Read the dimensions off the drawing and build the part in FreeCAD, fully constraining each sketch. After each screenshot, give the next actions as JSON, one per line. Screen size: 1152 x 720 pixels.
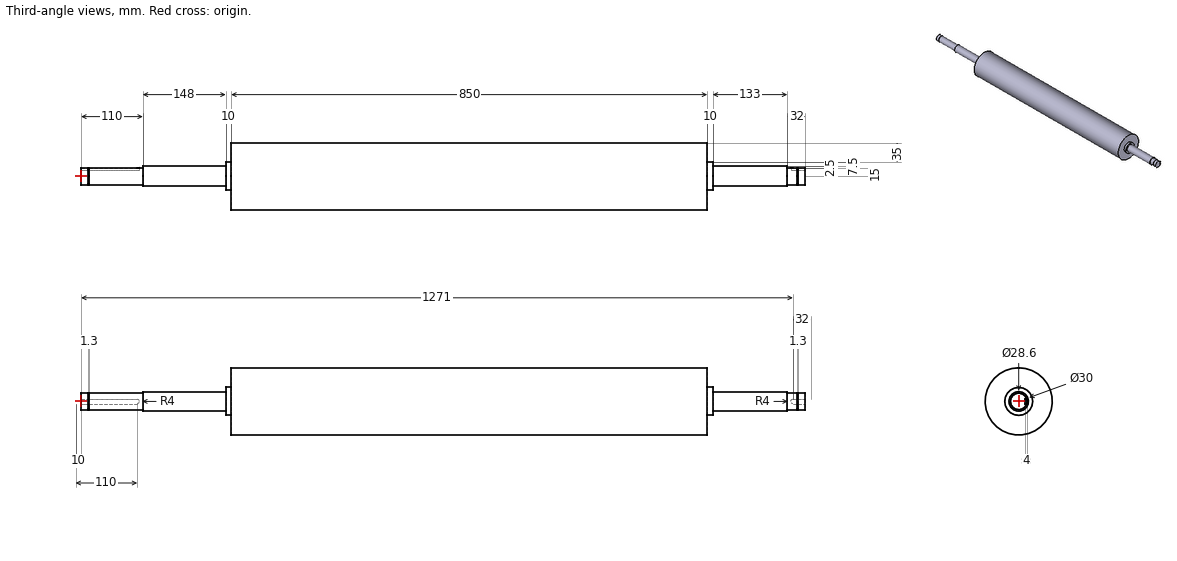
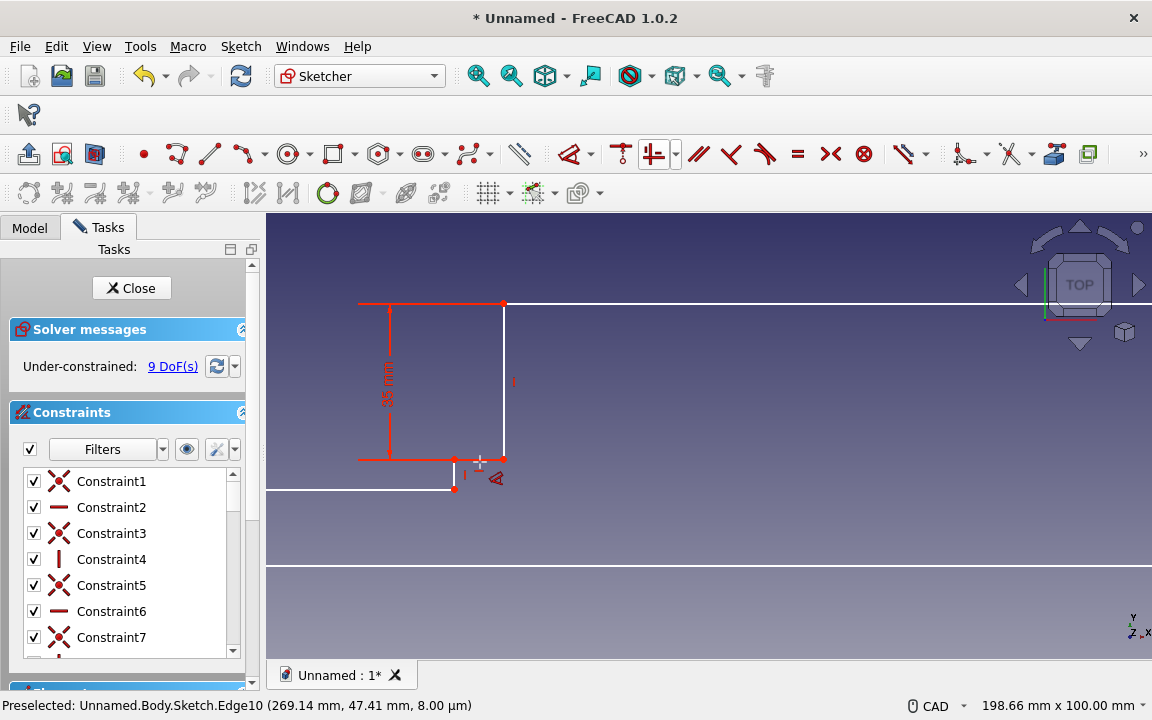
{"action": "left_click", "coordinate": [479, 460]}
{"action": "left_click", "coordinate": [479, 494]}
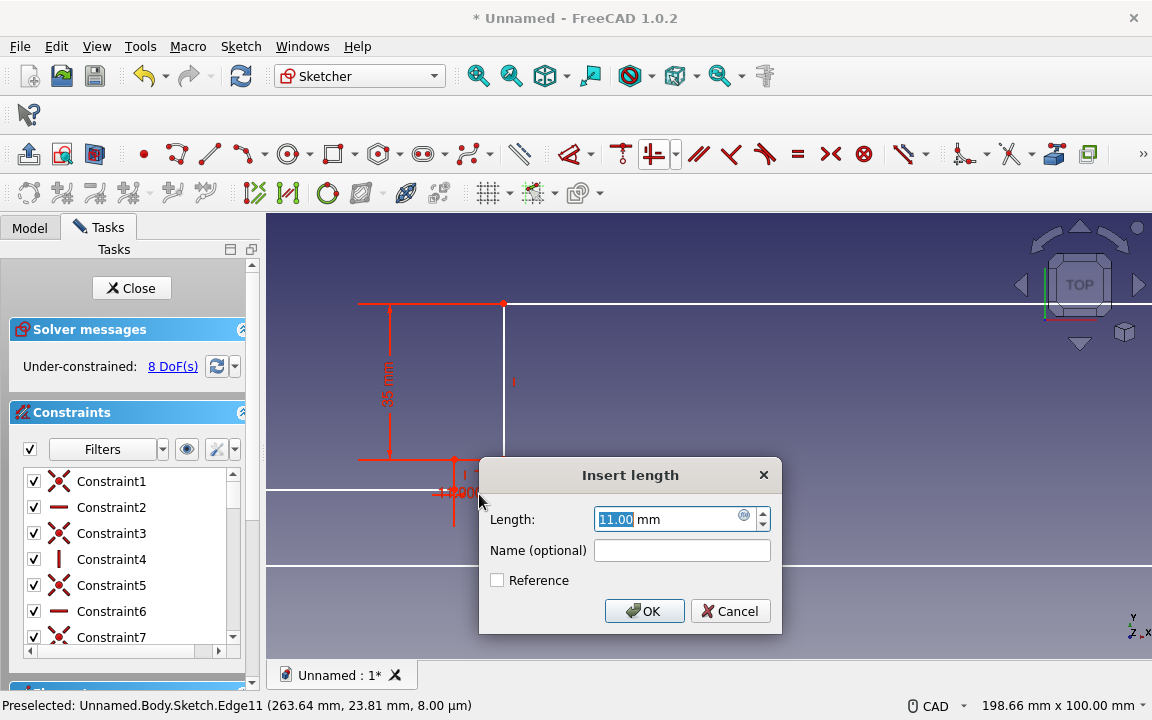
{"action": "type", "text": "10"}
{"action": "key", "text": "Return"}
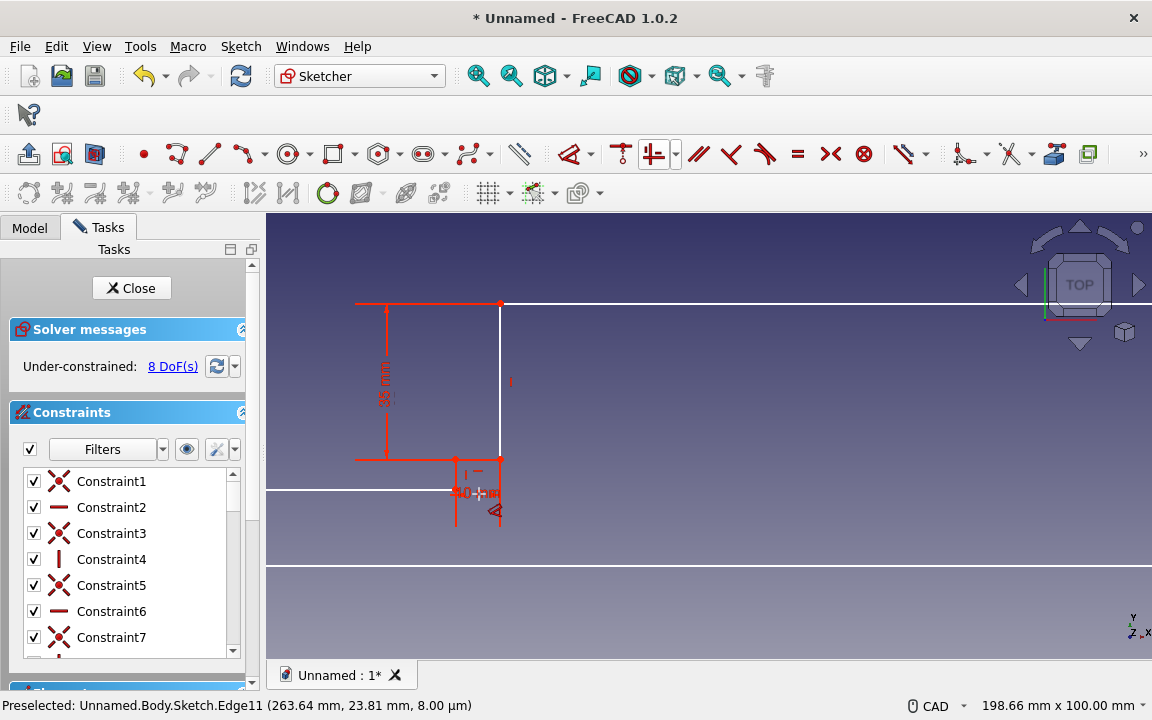
{"action": "scroll", "coordinate": [486, 436], "scroll_direction": "down", "scroll_amount": 12}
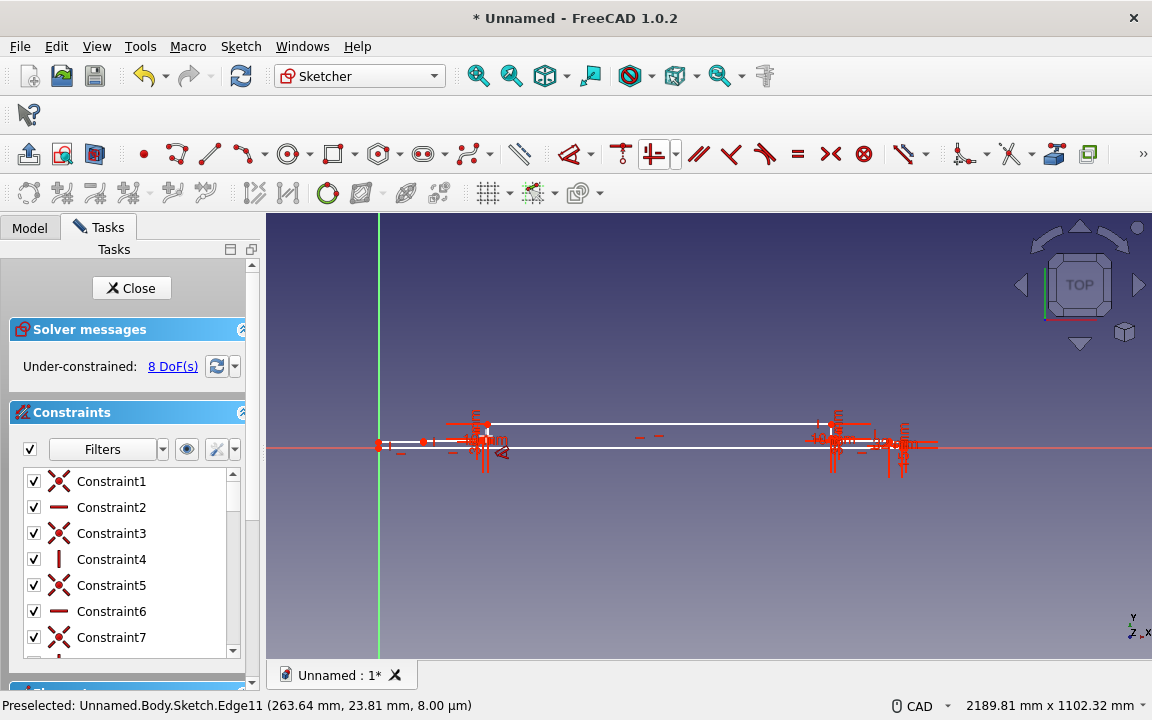
{"action": "scroll", "coordinate": [379, 444], "scroll_direction": "up", "scroll_amount": 11}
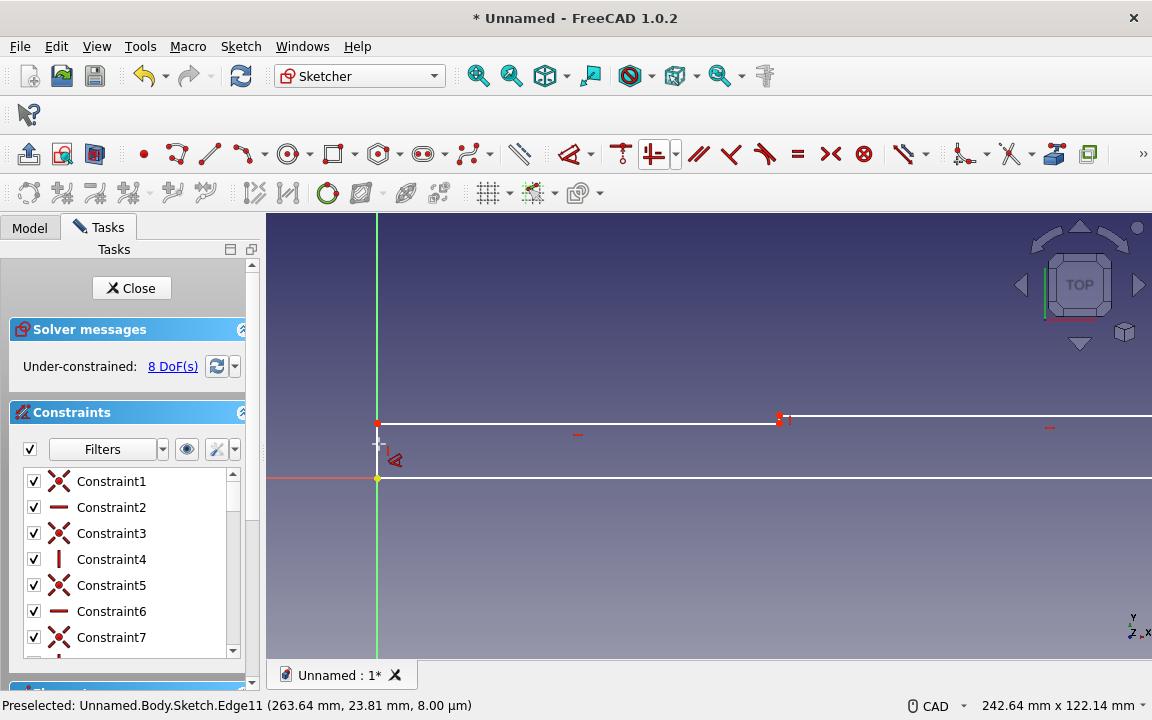
{"action": "left_click", "coordinate": [377, 440]}
{"action": "left_click", "coordinate": [343, 451]}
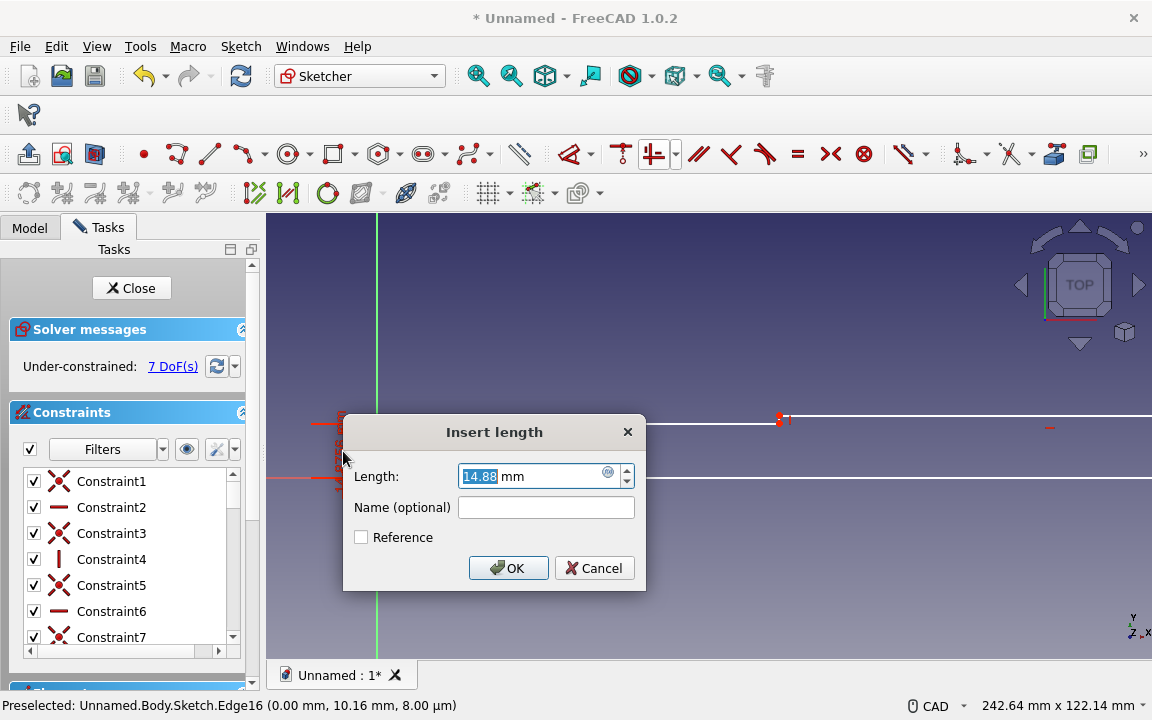
{"action": "type", "text": "15"}
{"action": "key", "text": "Return"}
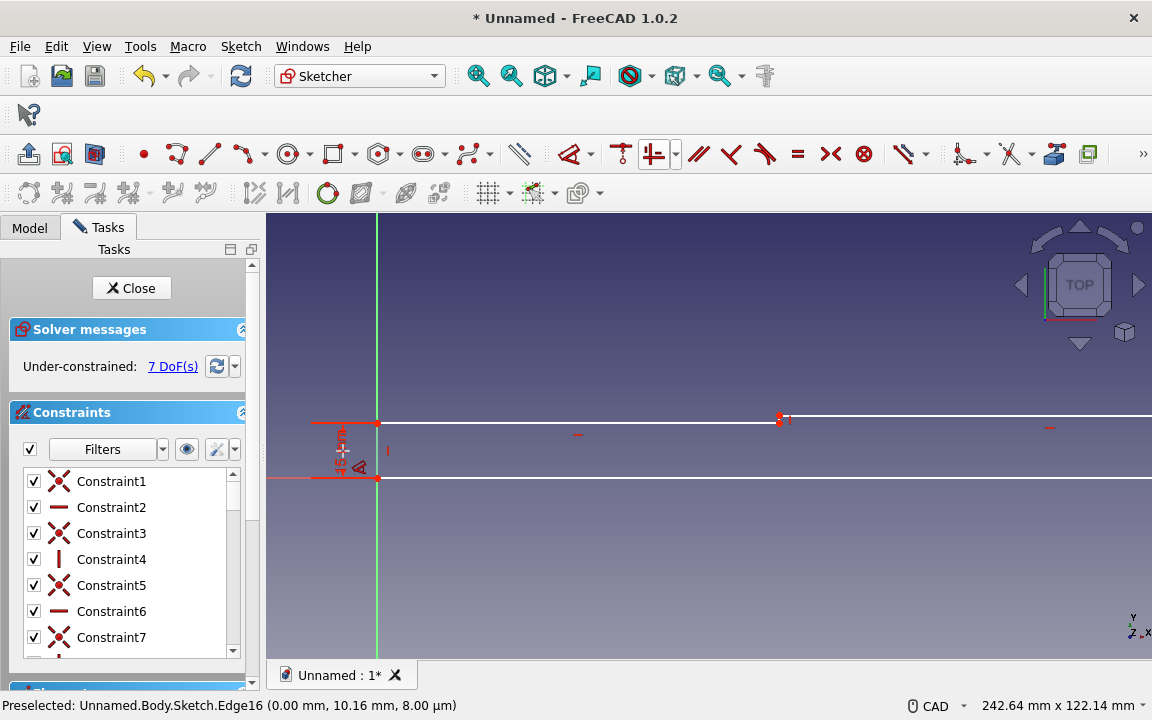
{"action": "scroll", "coordinate": [379, 444], "scroll_direction": "down", "scroll_amount": 11}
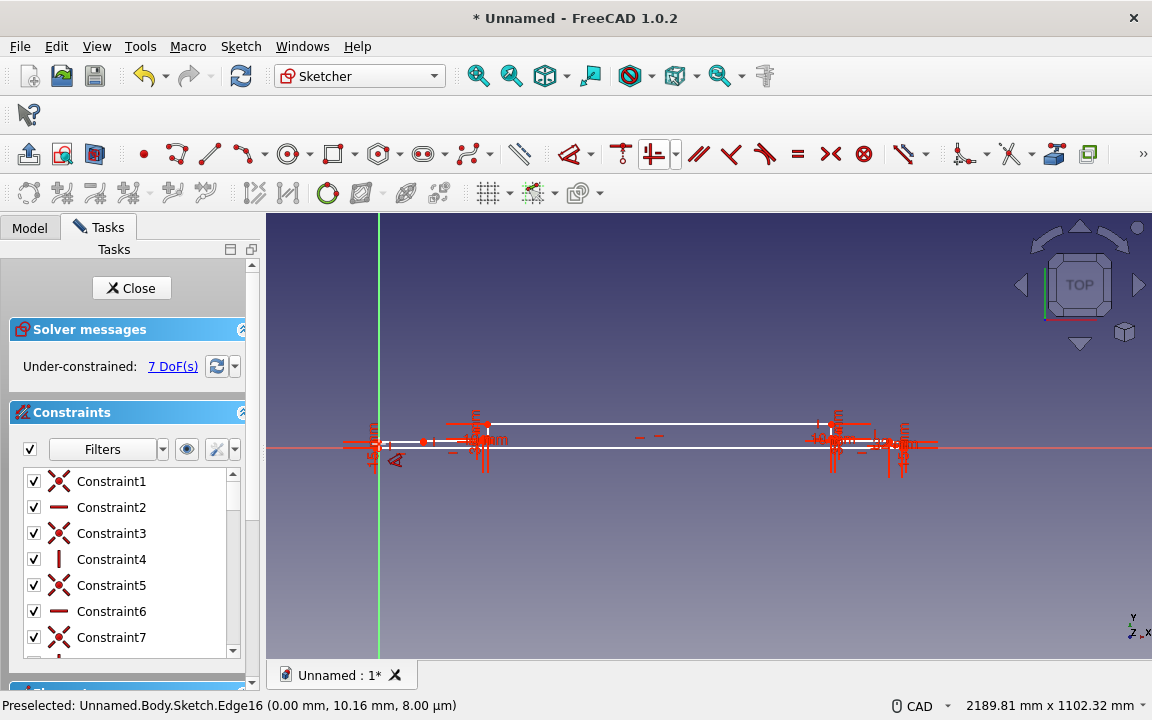
{"action": "scroll", "coordinate": [889, 442], "scroll_direction": "up", "scroll_amount": 19}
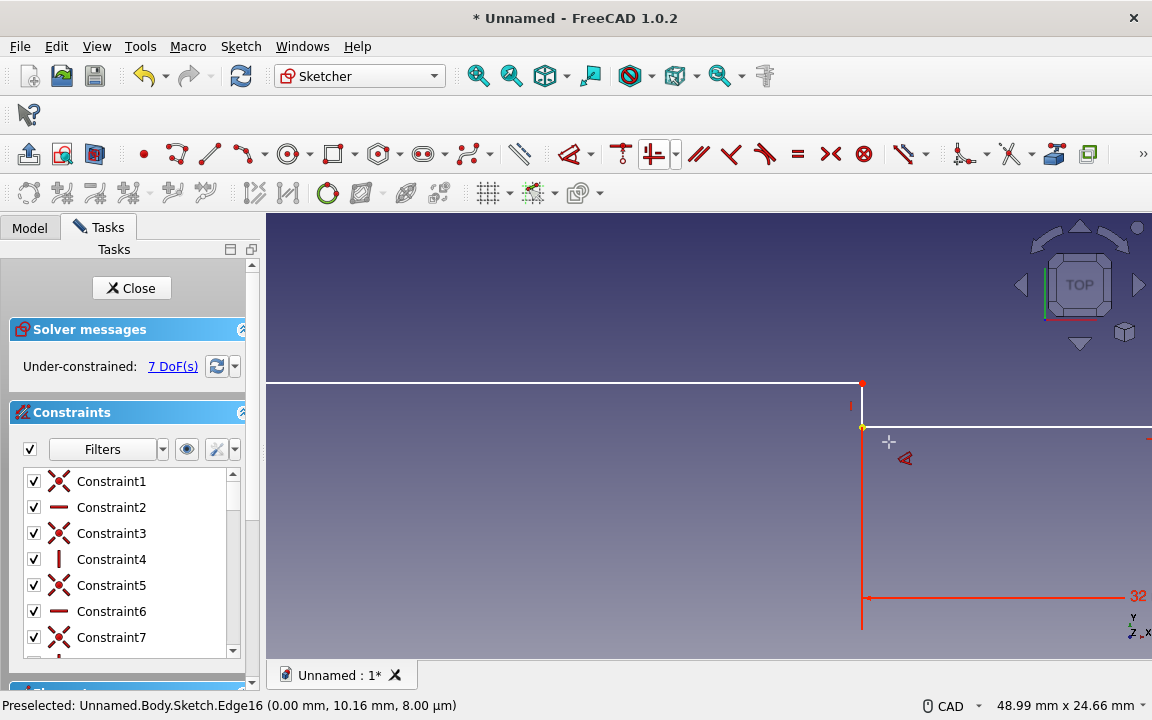
{"action": "left_click", "coordinate": [862, 405]}
{"action": "left_click", "coordinate": [896, 405]}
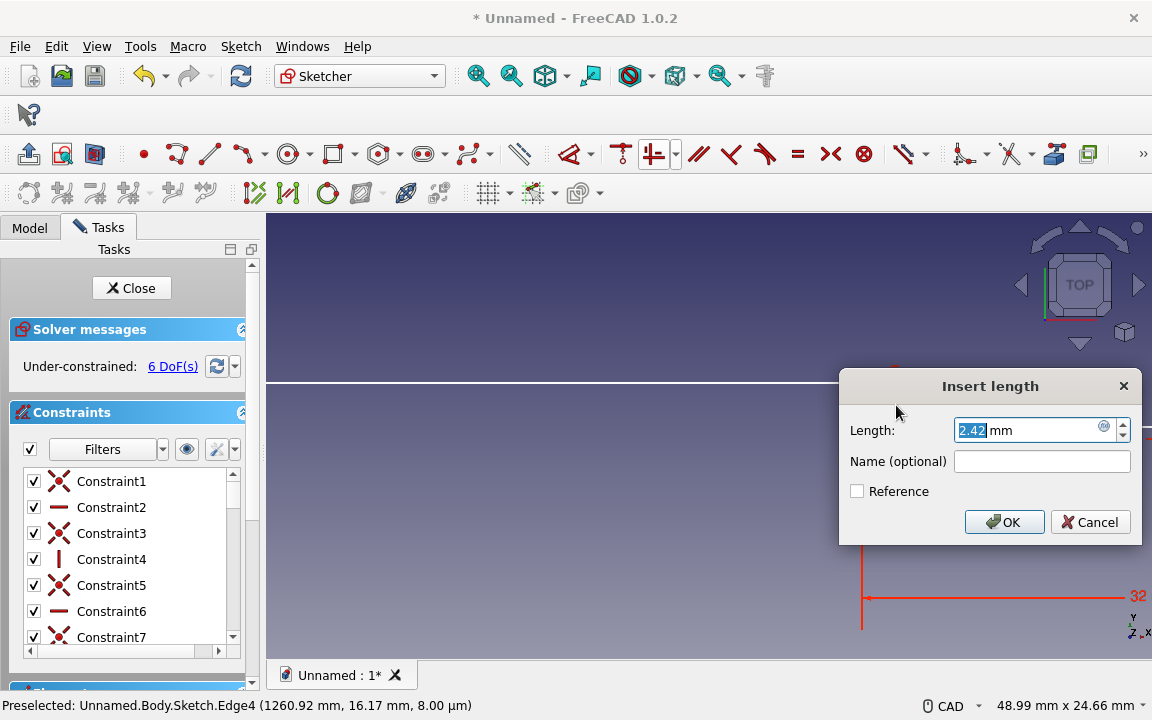
{"action": "type", "text": "2.5"}
{"action": "key", "text": "Return"}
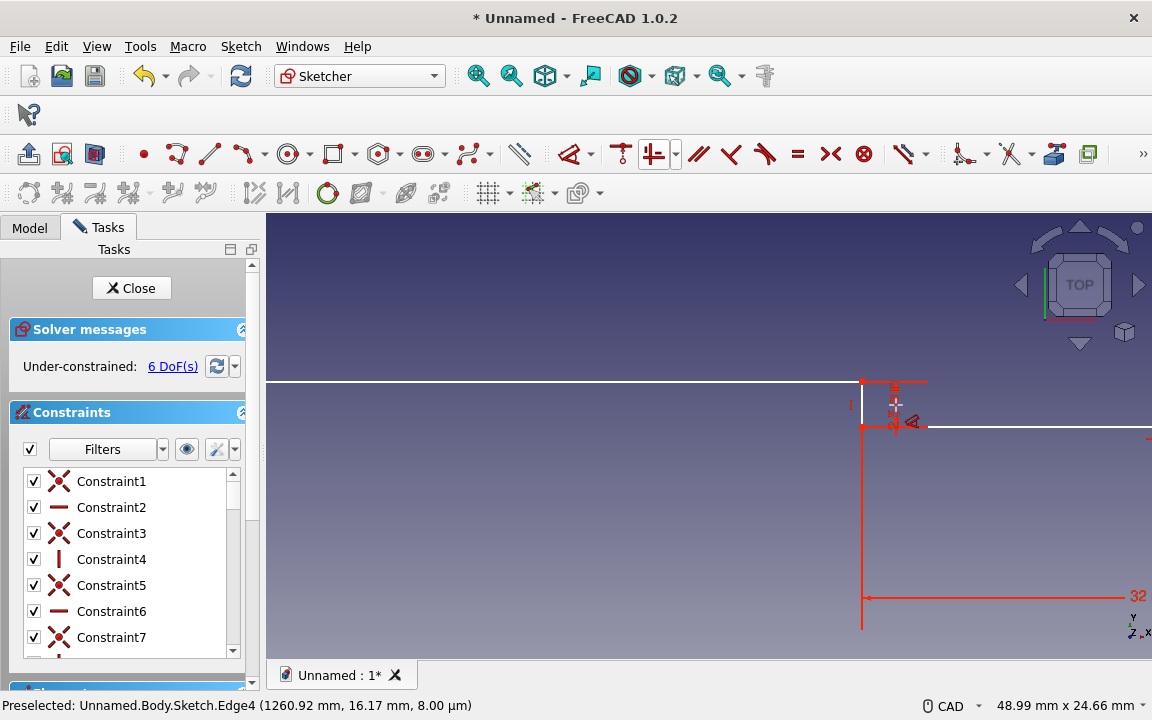
{"action": "scroll", "coordinate": [946, 444], "scroll_direction": "down", "scroll_amount": 18}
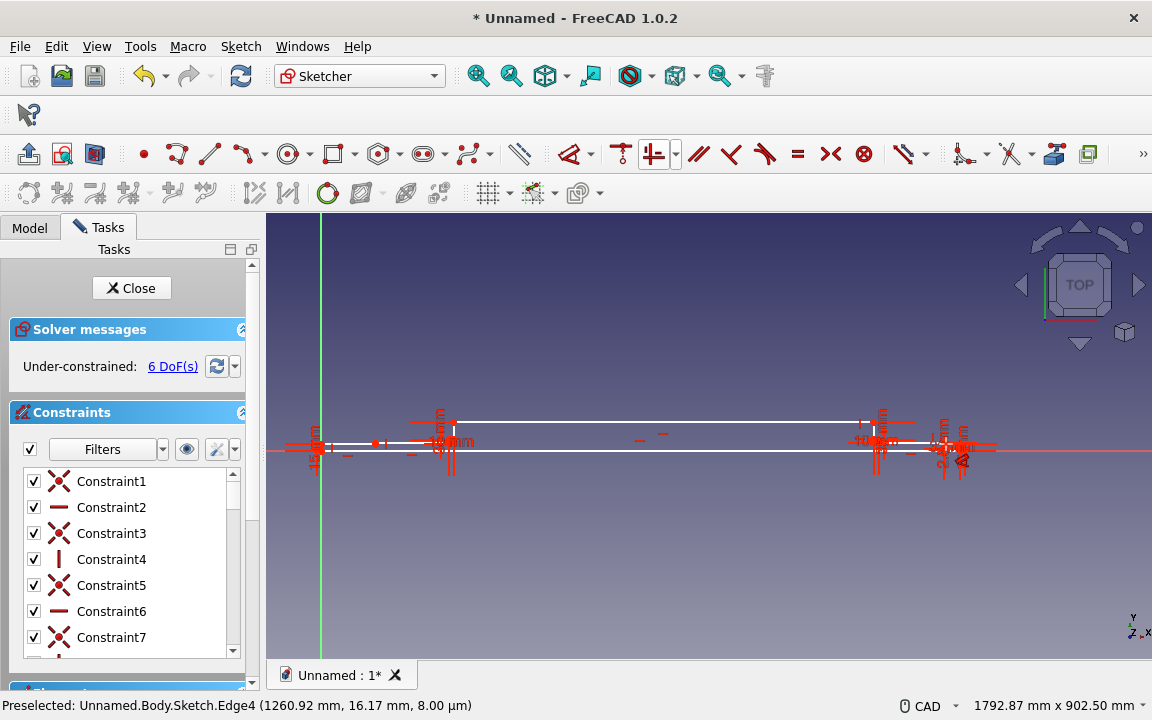
{"action": "scroll", "coordinate": [931, 443], "scroll_direction": "up", "scroll_amount": 3}